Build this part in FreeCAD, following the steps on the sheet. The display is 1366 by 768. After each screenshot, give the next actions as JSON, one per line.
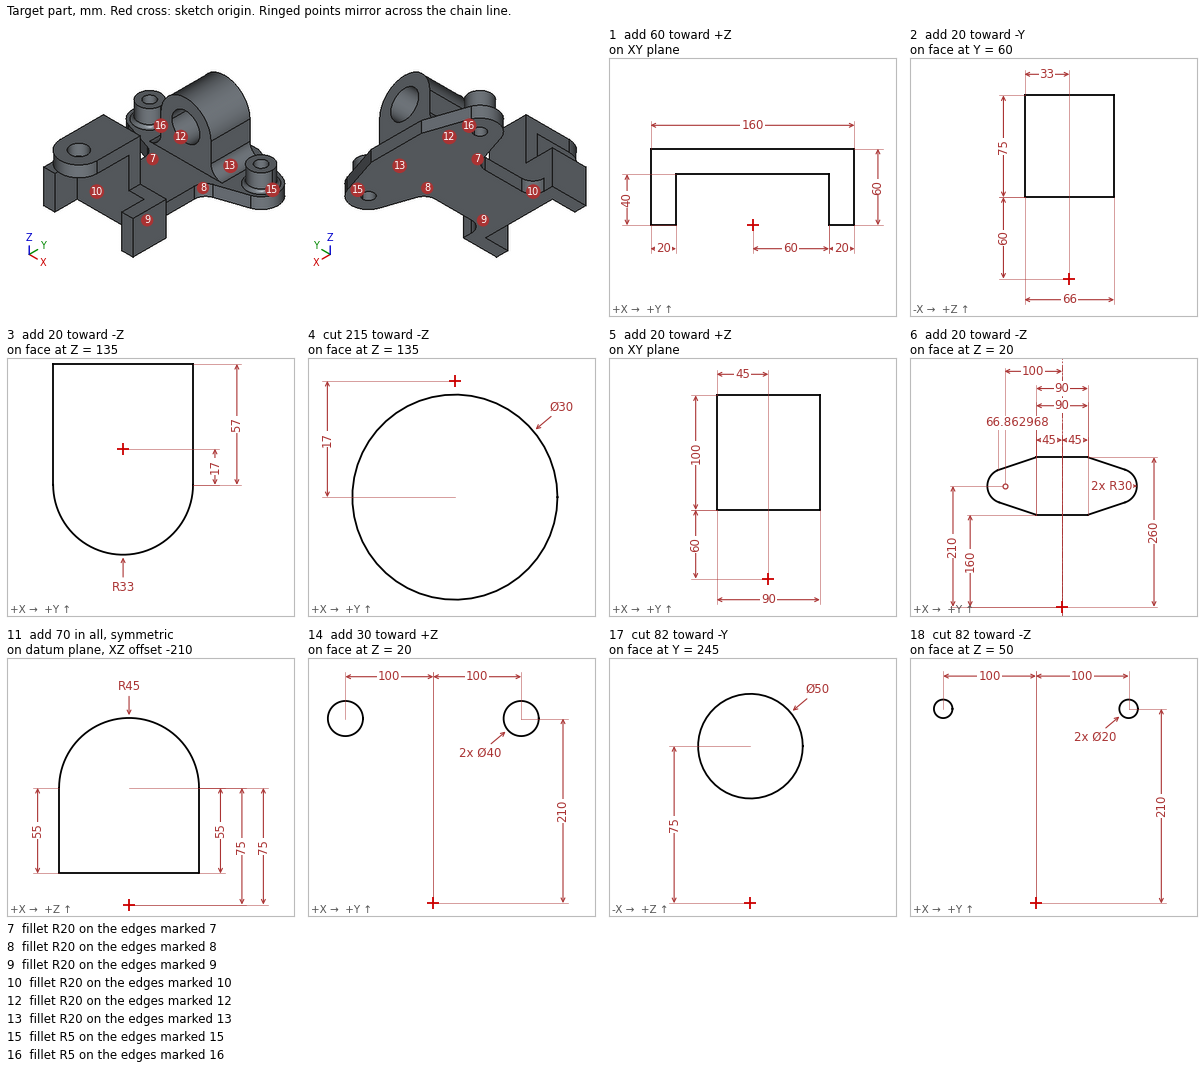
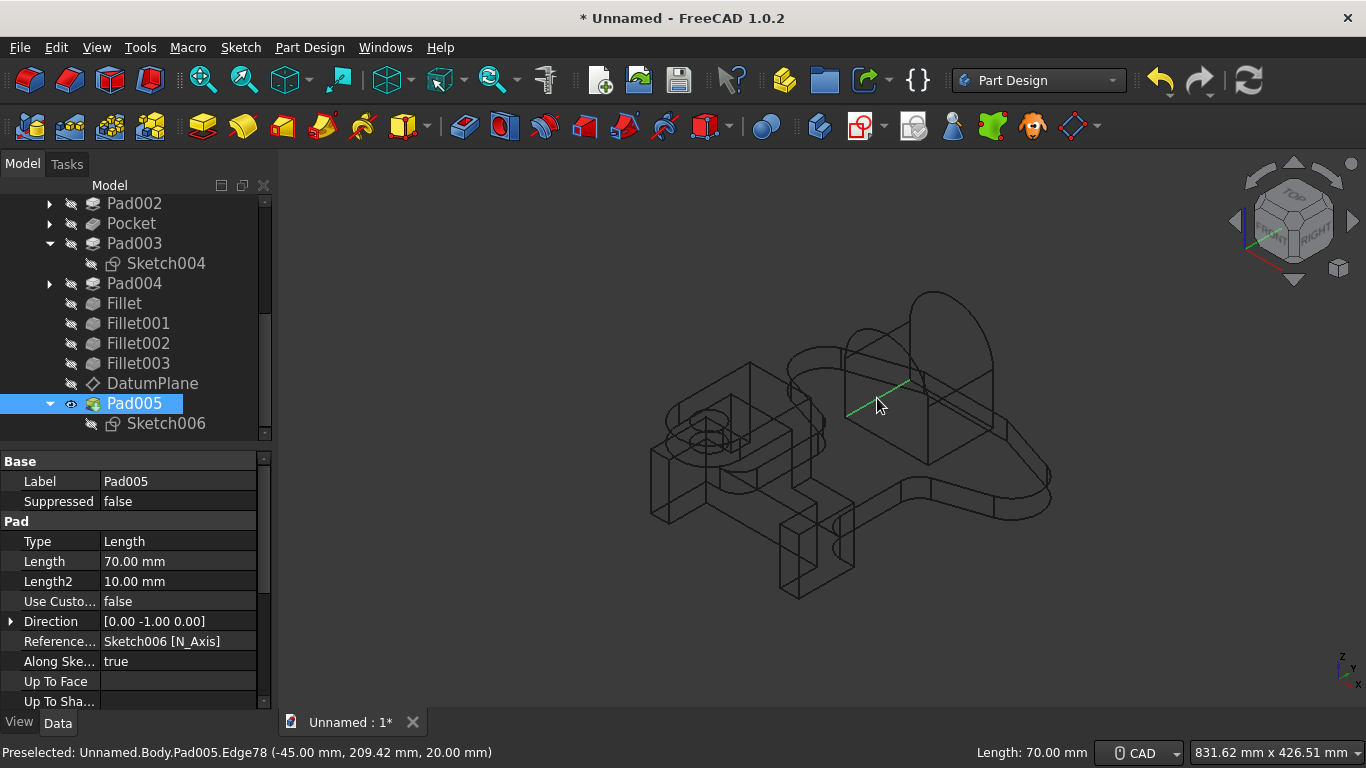
{"action": "key", "text": "v 1"}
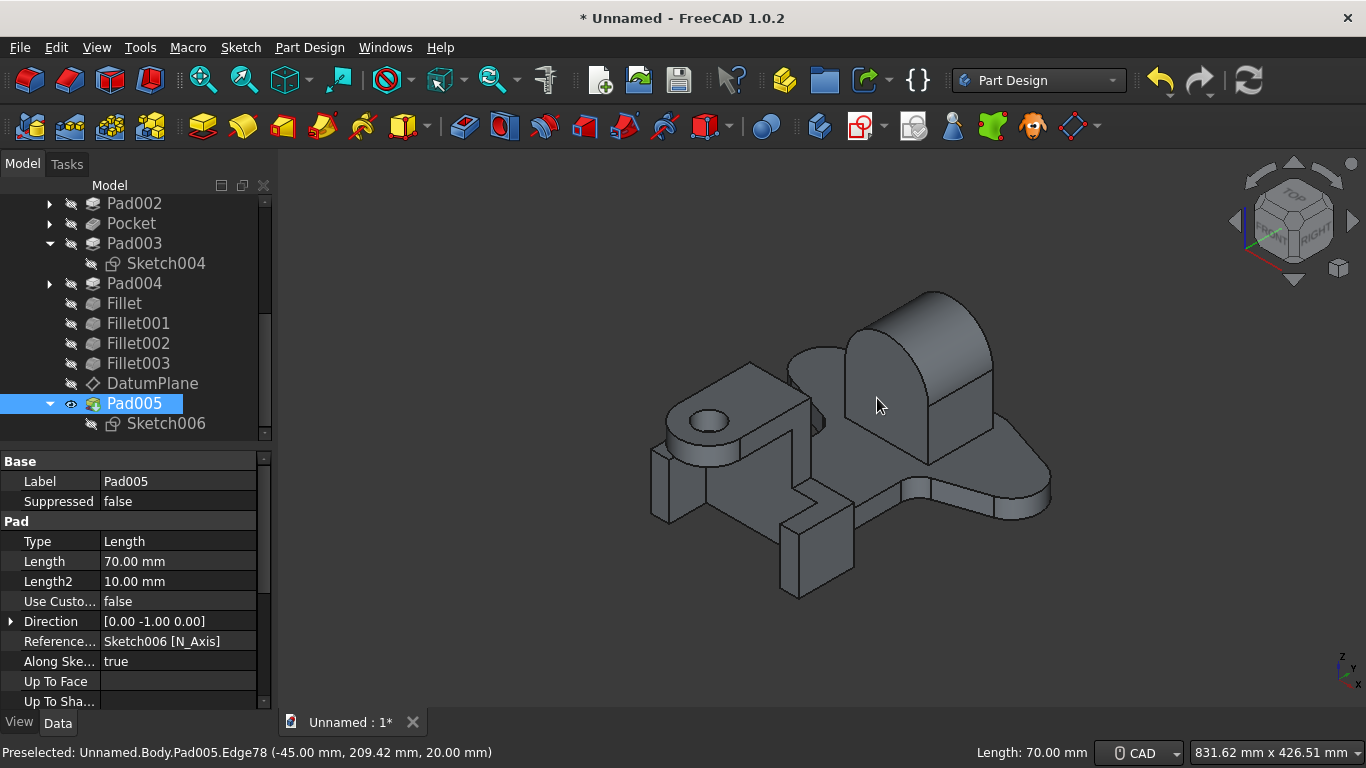
{"action": "left_click", "coordinate": [30, 80]}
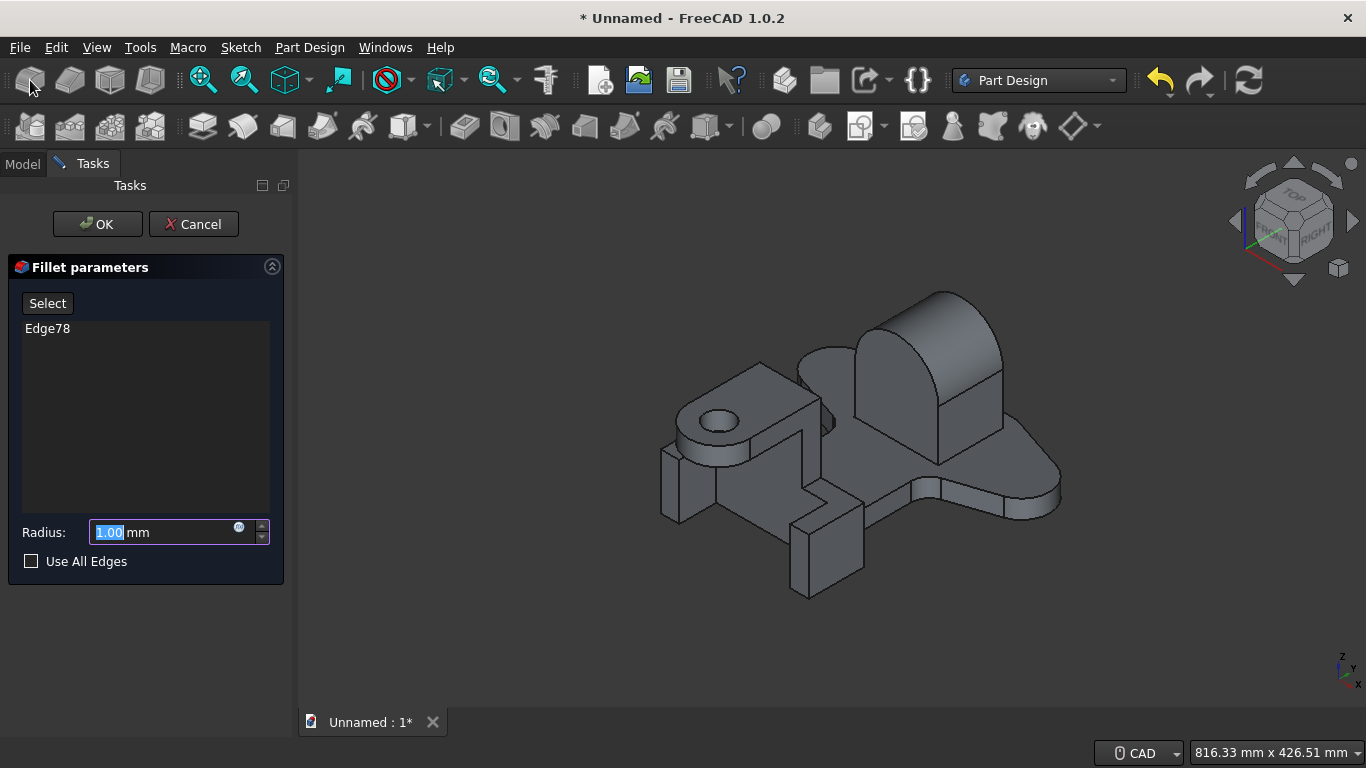
{"action": "type", "text": "20"}
{"action": "key", "text": "Tab"}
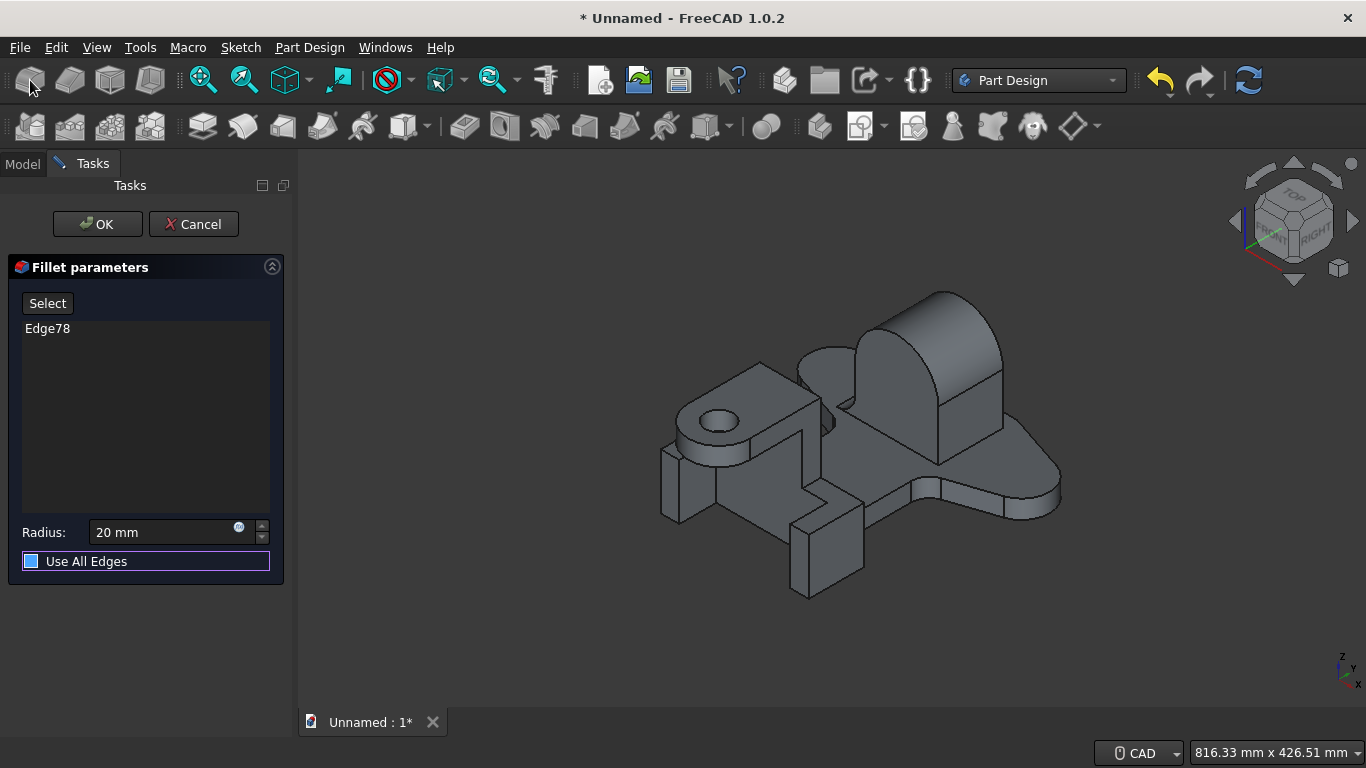
{"action": "left_click", "coordinate": [98, 224]}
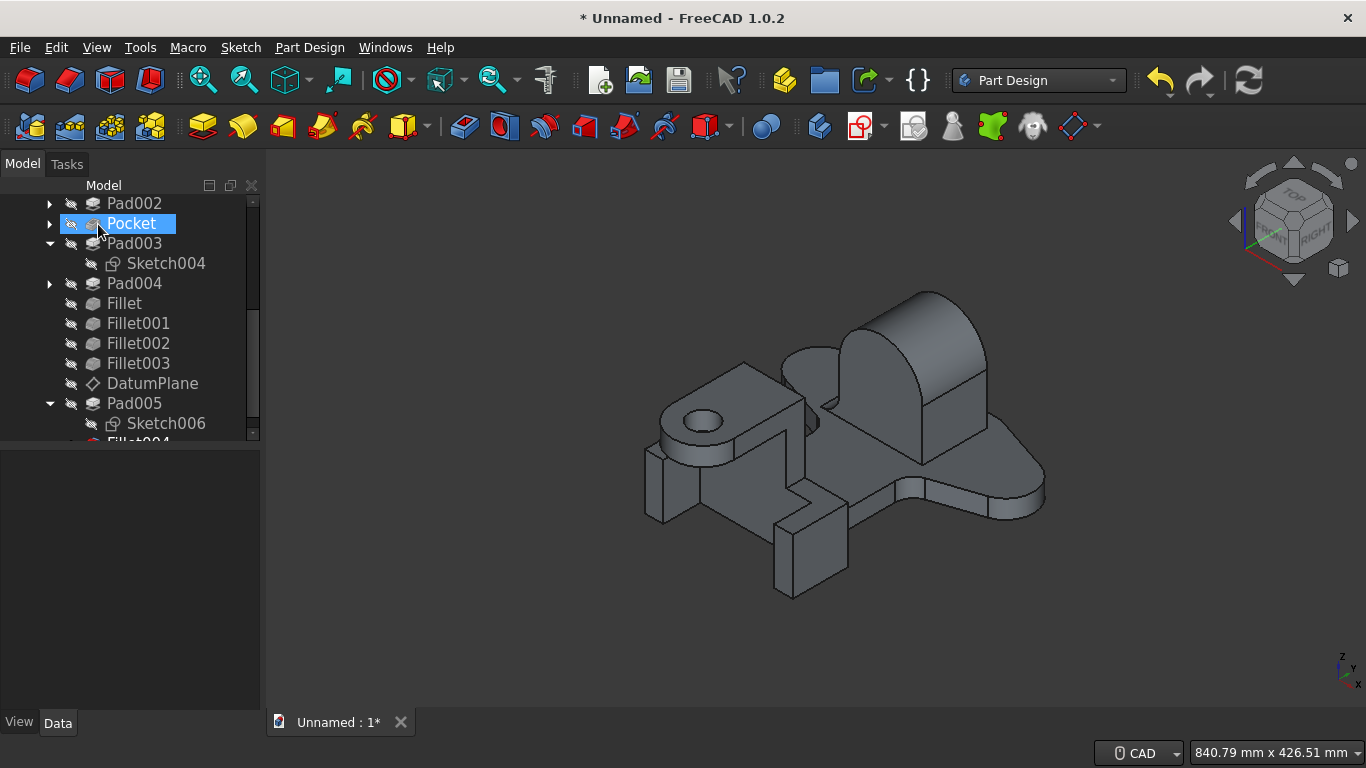
{"action": "key", "text": "2"}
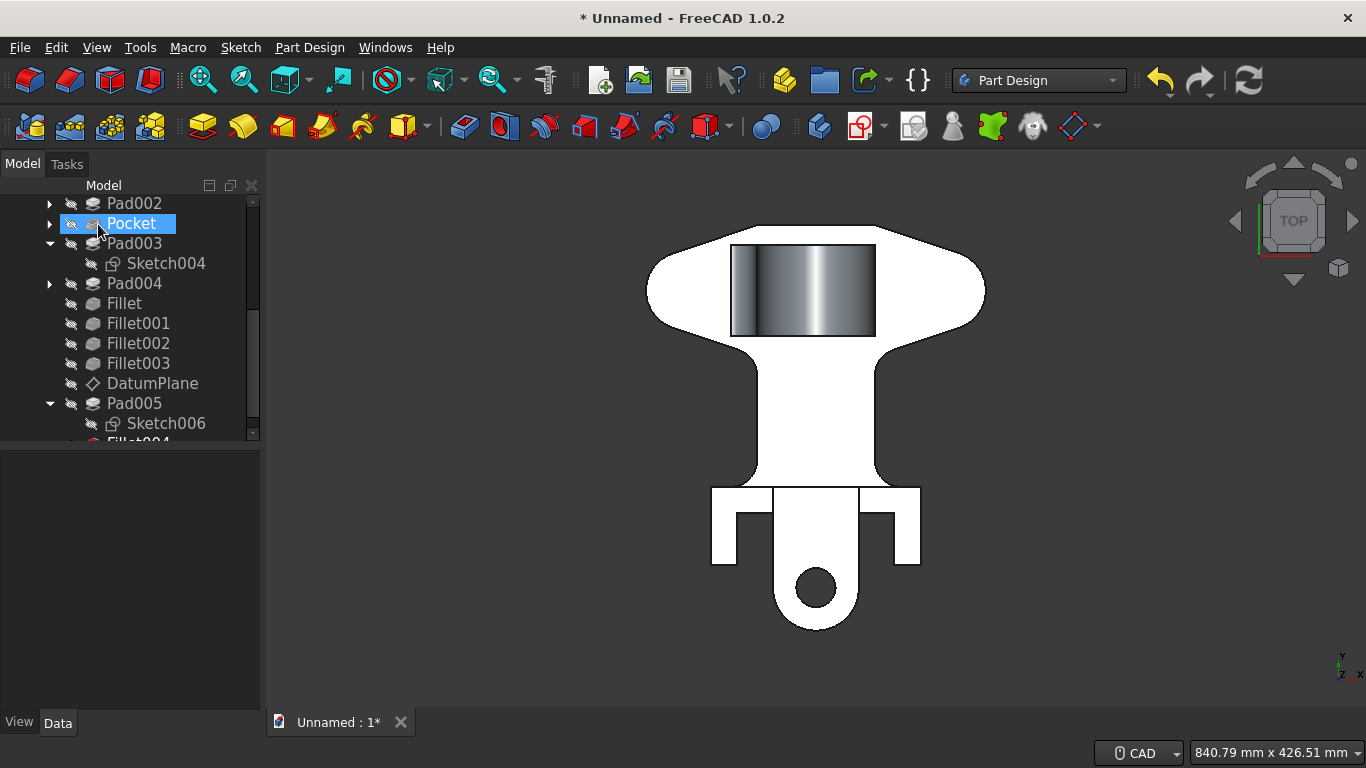
{"action": "key", "text": "0"}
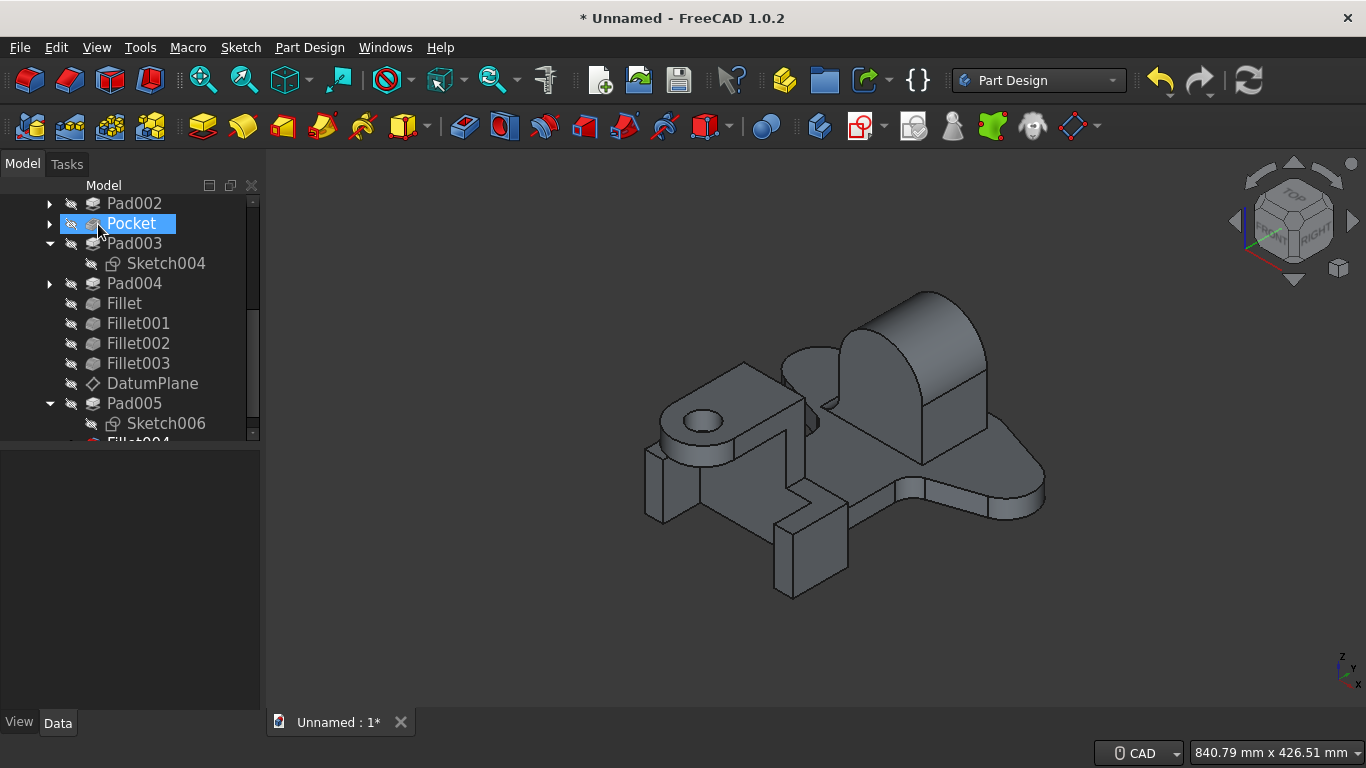
{"action": "key", "text": "1"}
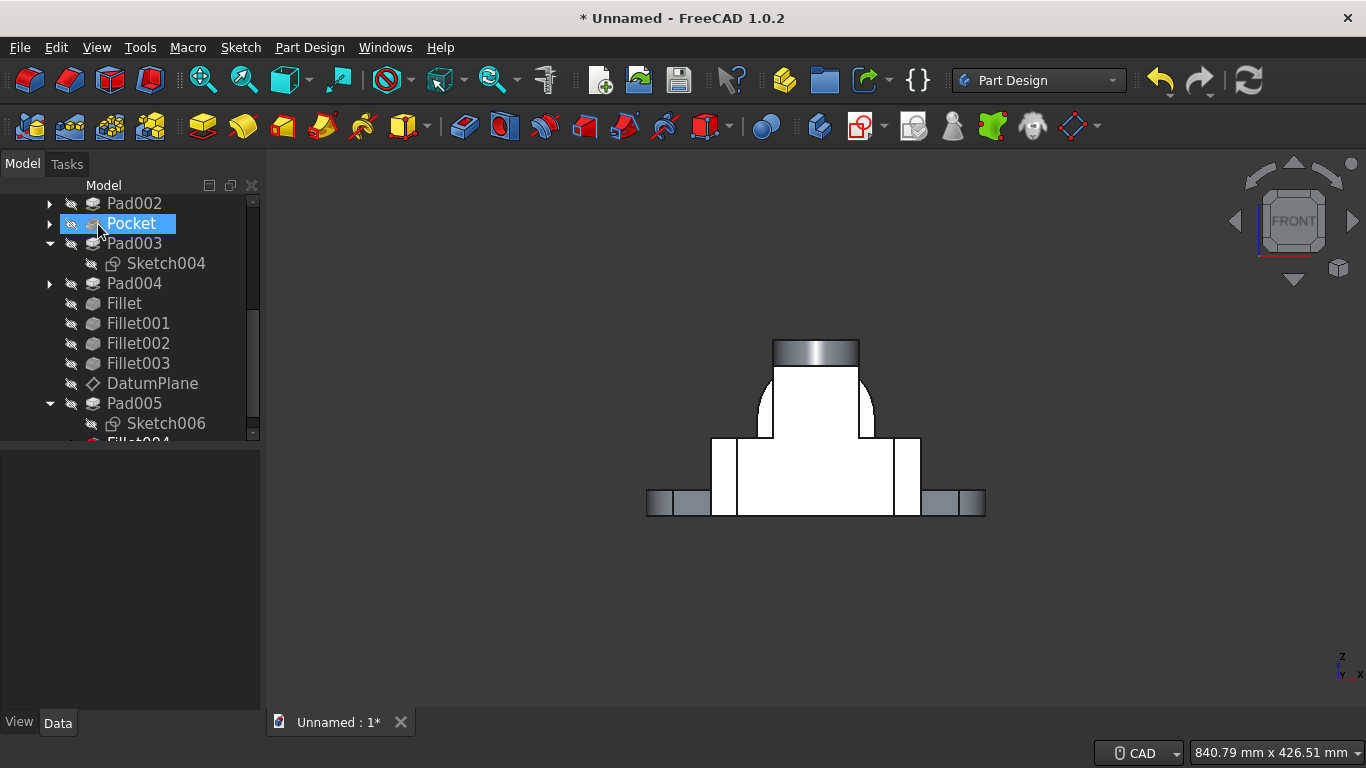
{"action": "key", "text": "v f"}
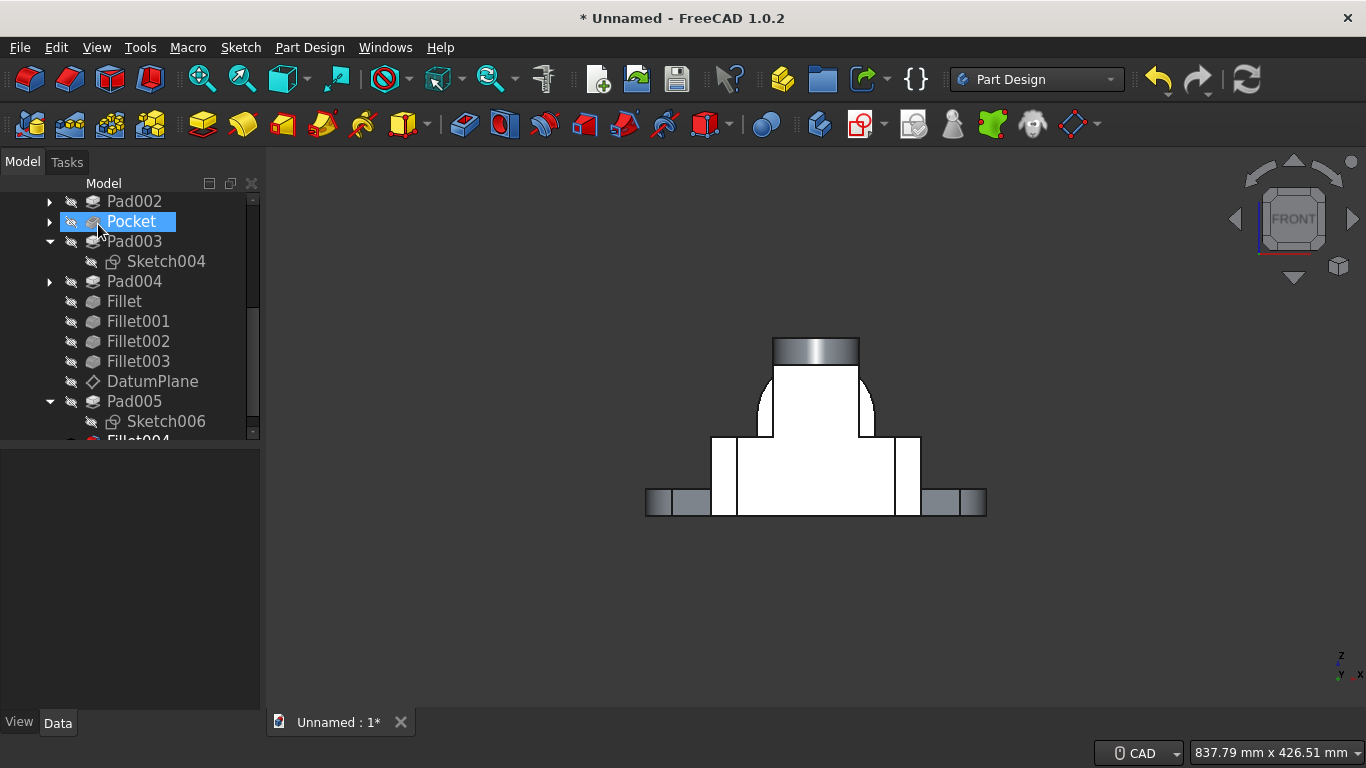
{"action": "key", "text": "3"}